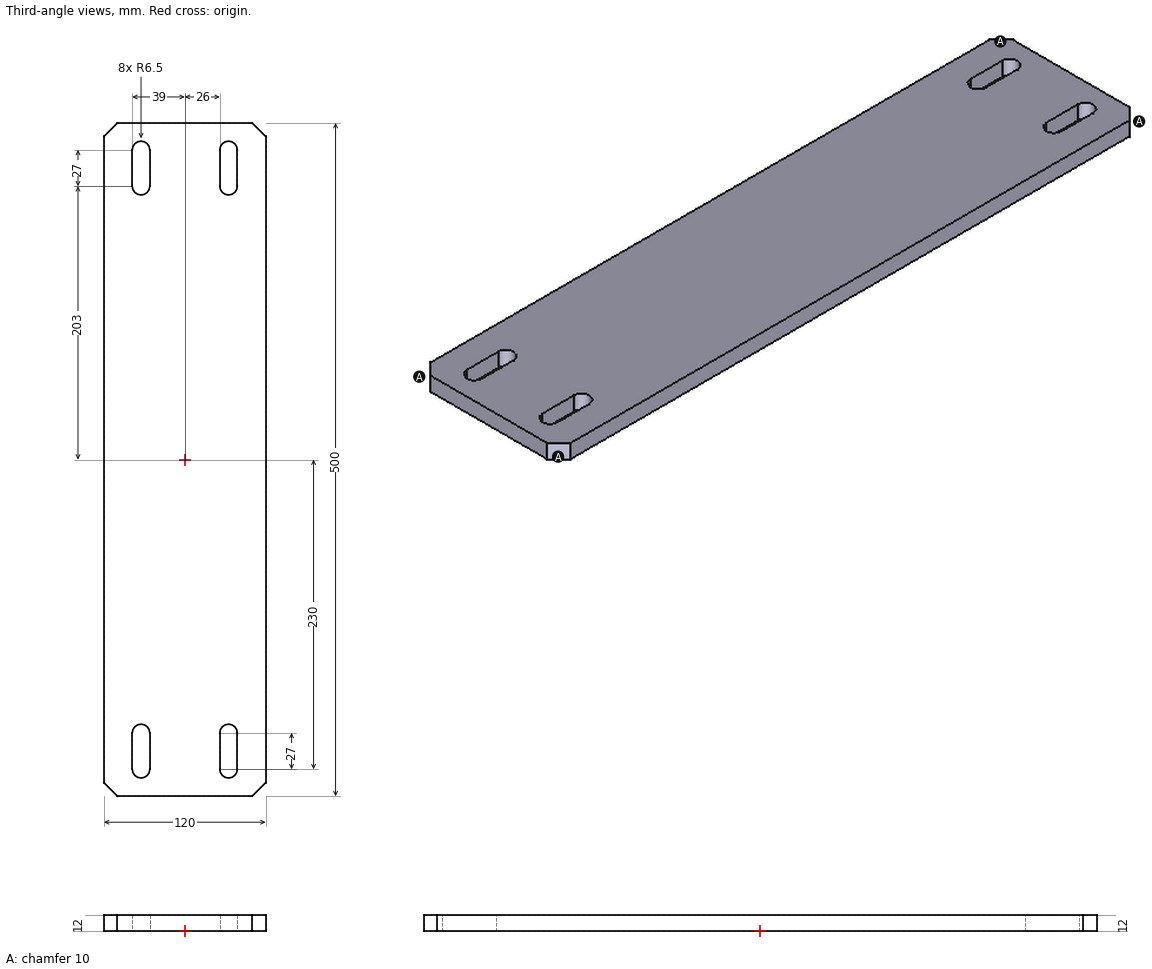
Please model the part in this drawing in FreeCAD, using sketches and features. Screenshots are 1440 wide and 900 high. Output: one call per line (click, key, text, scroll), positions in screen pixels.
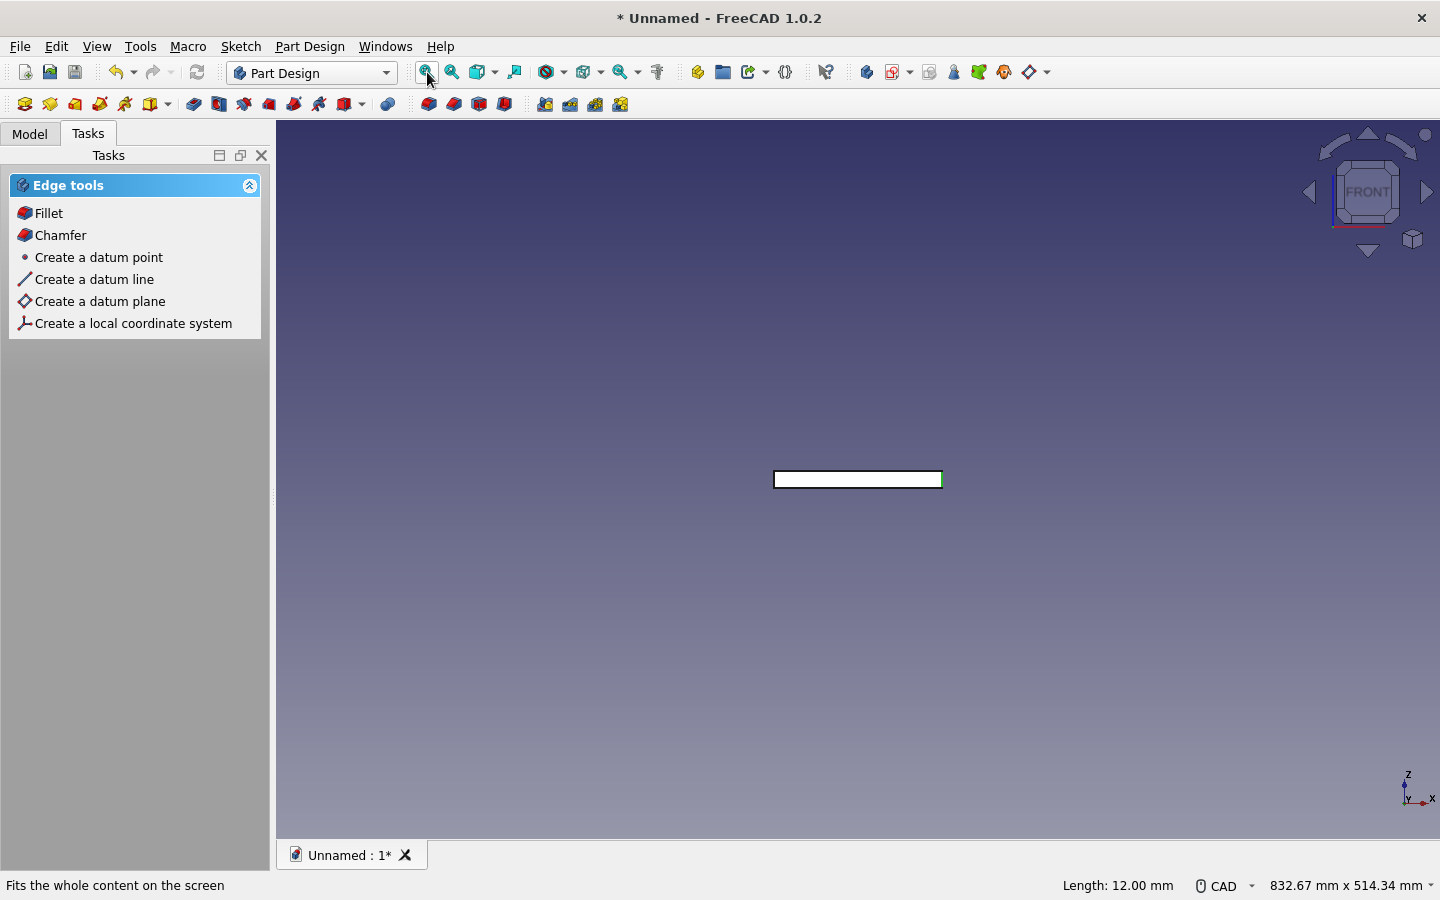
click(774, 479, ctrl)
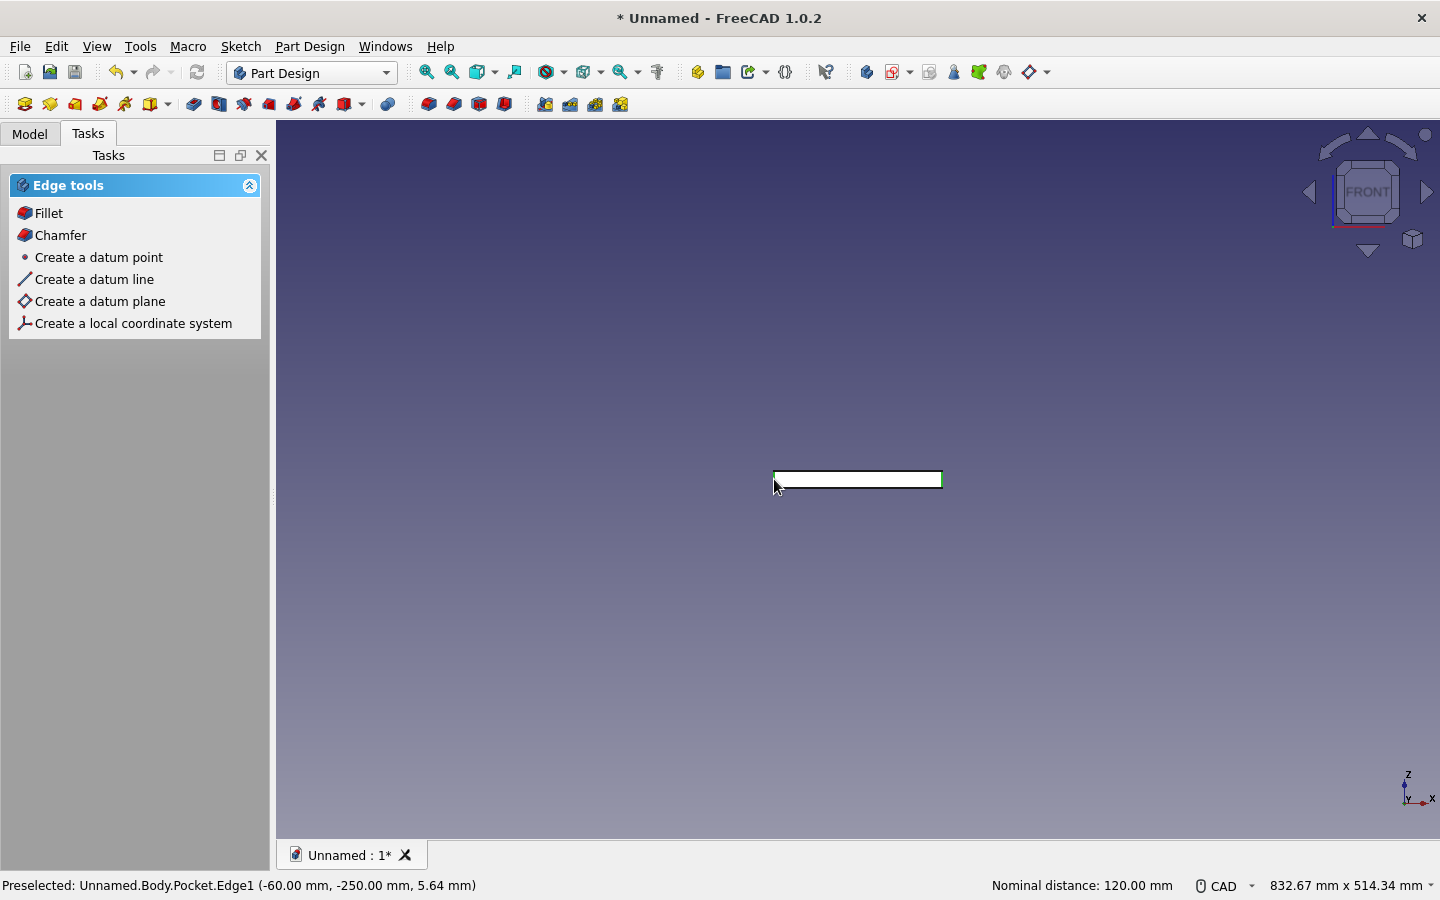
scroll(774, 479, up, 5)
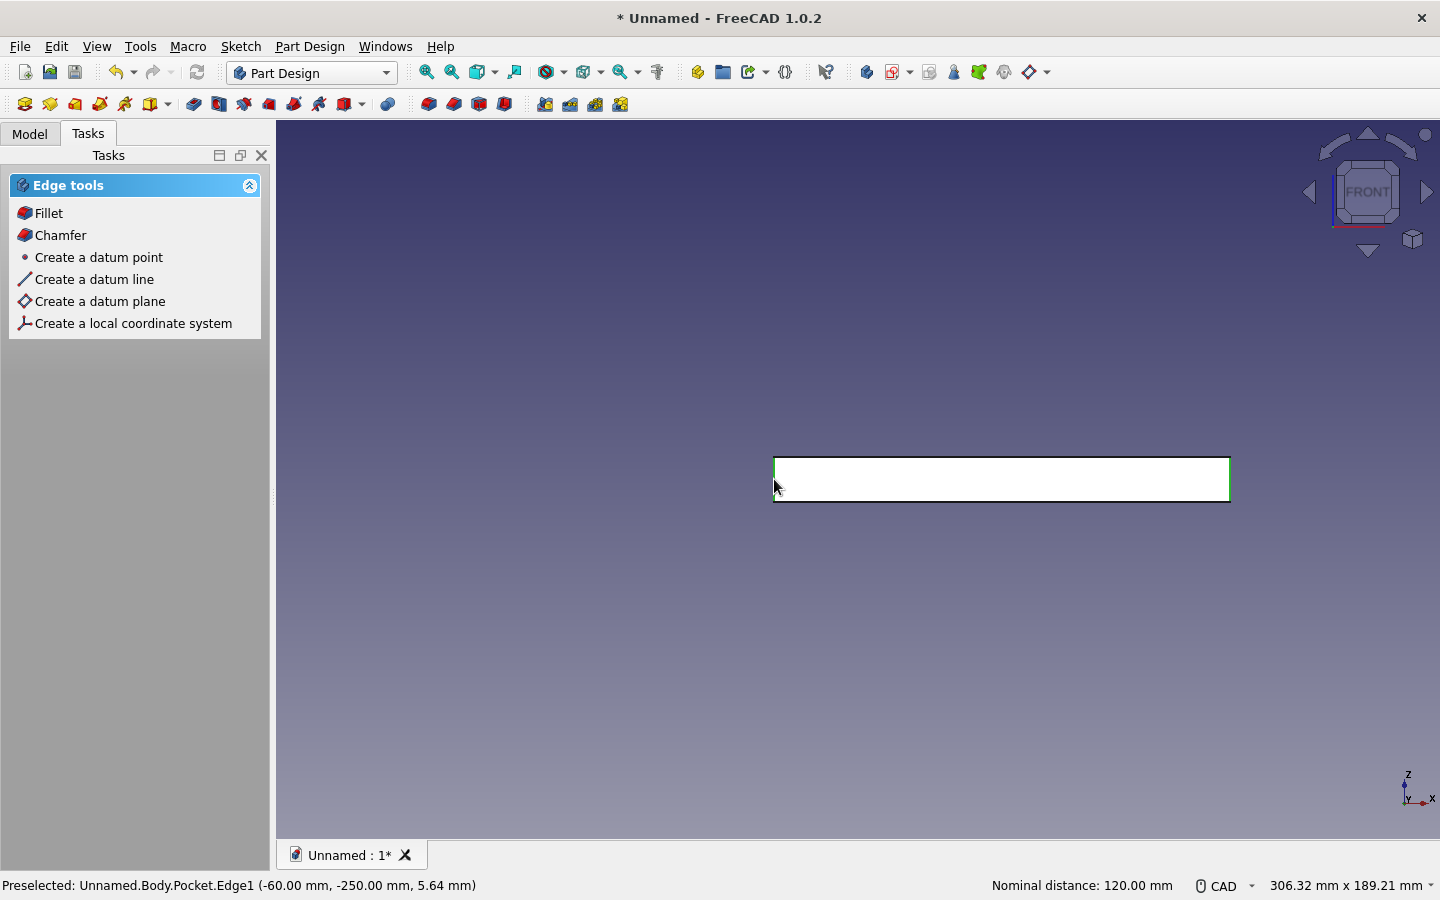
key(v)
key(f)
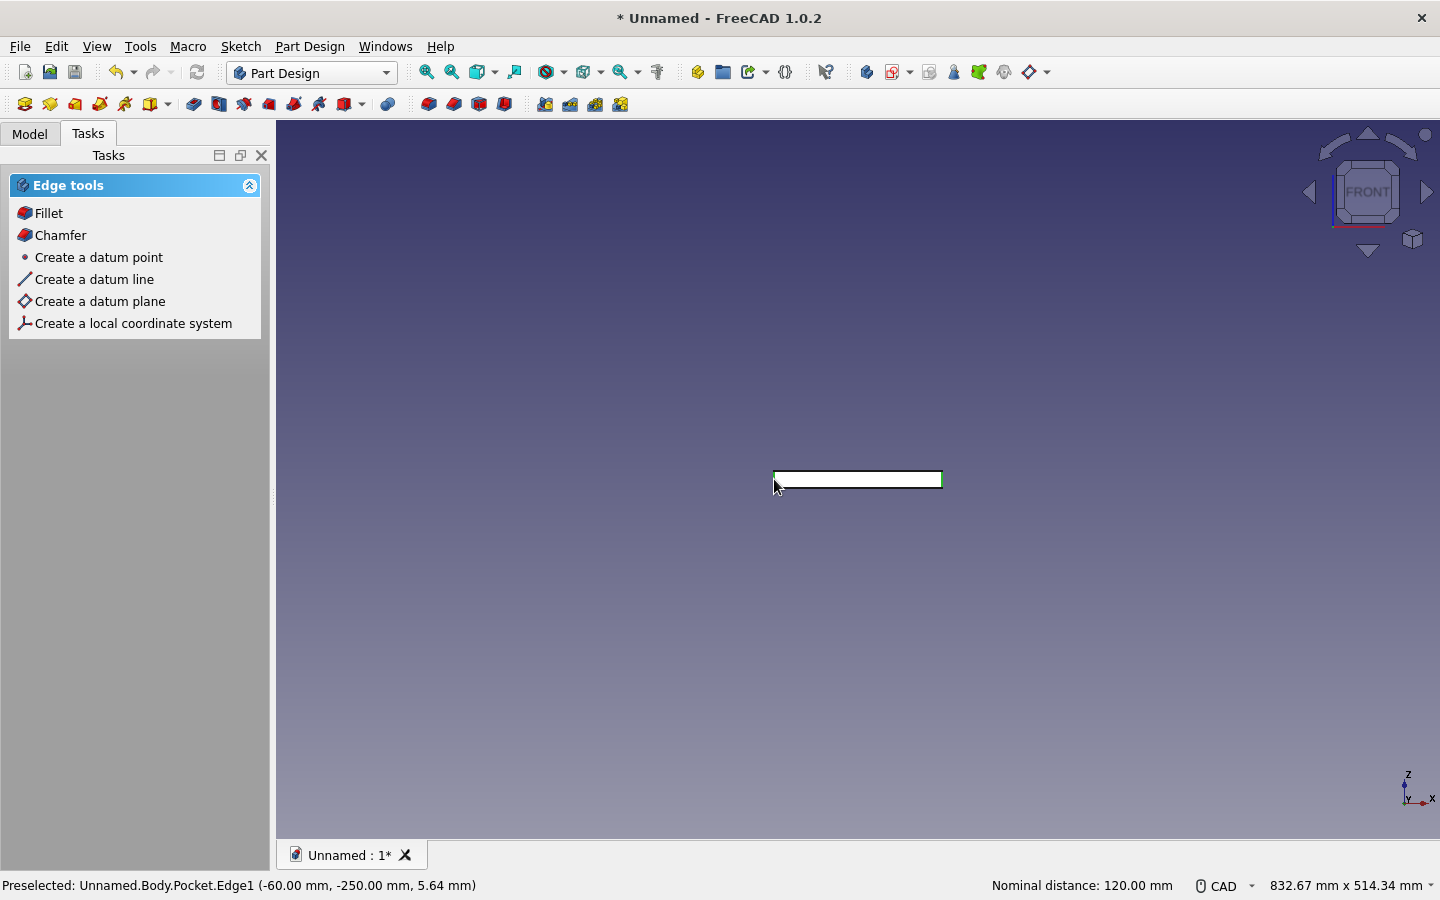
key(3)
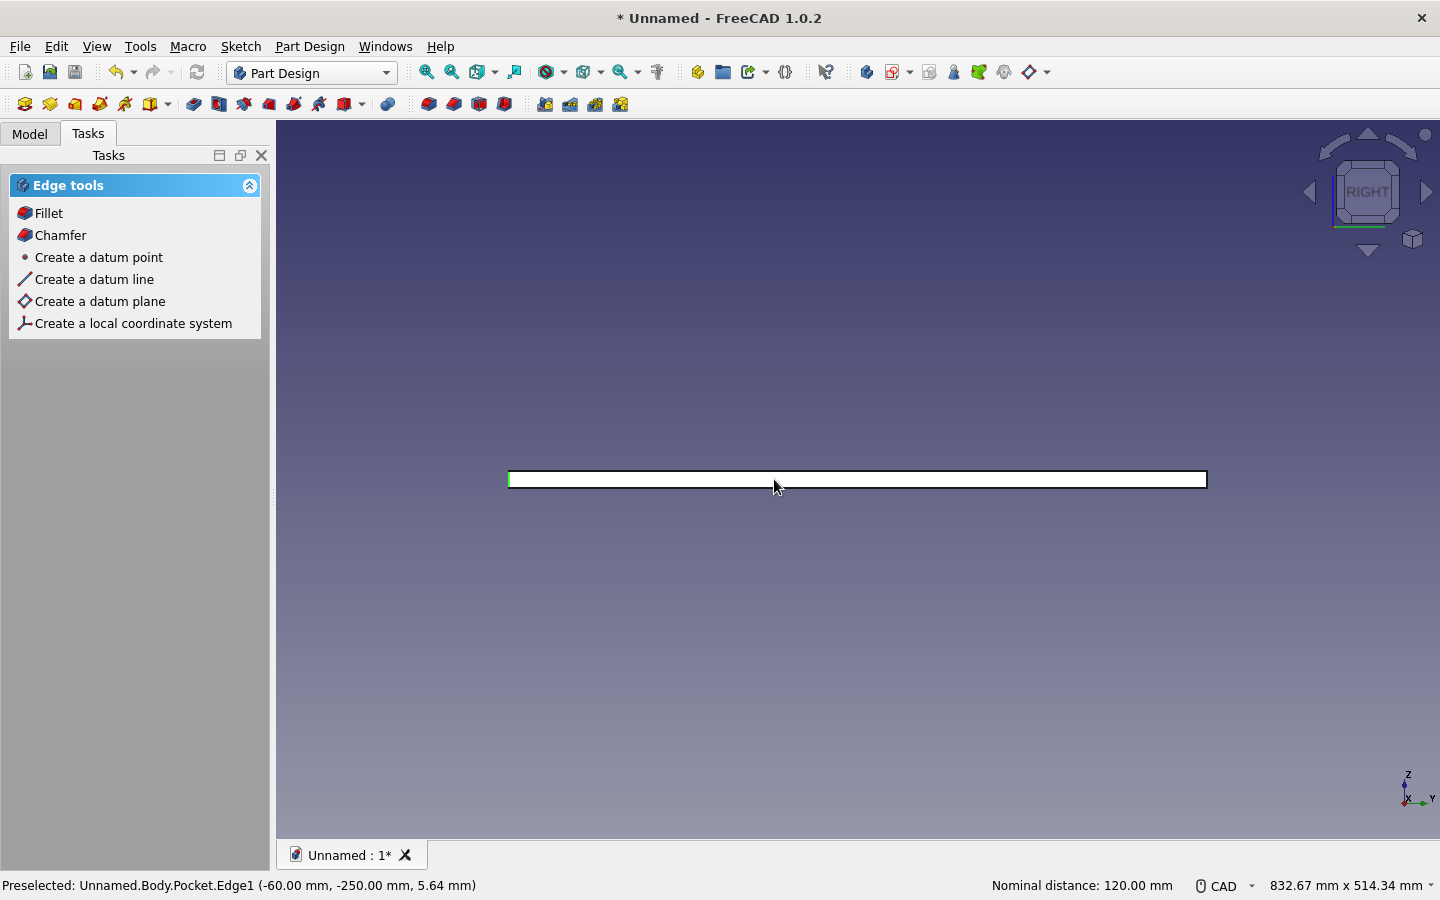
click(1207, 478, ctrl)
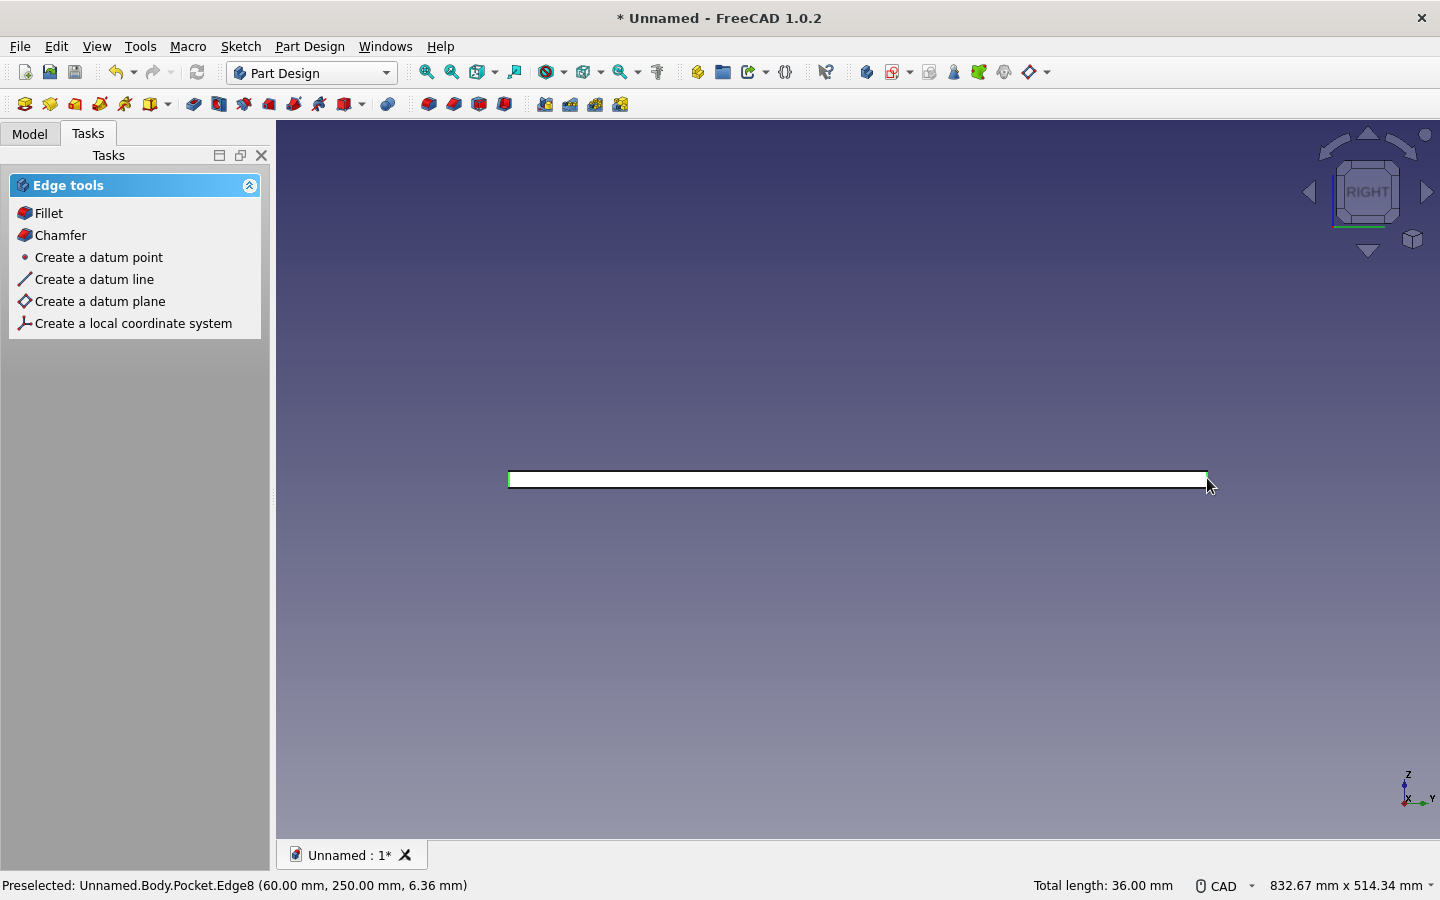
scroll(1207, 478, up, 5)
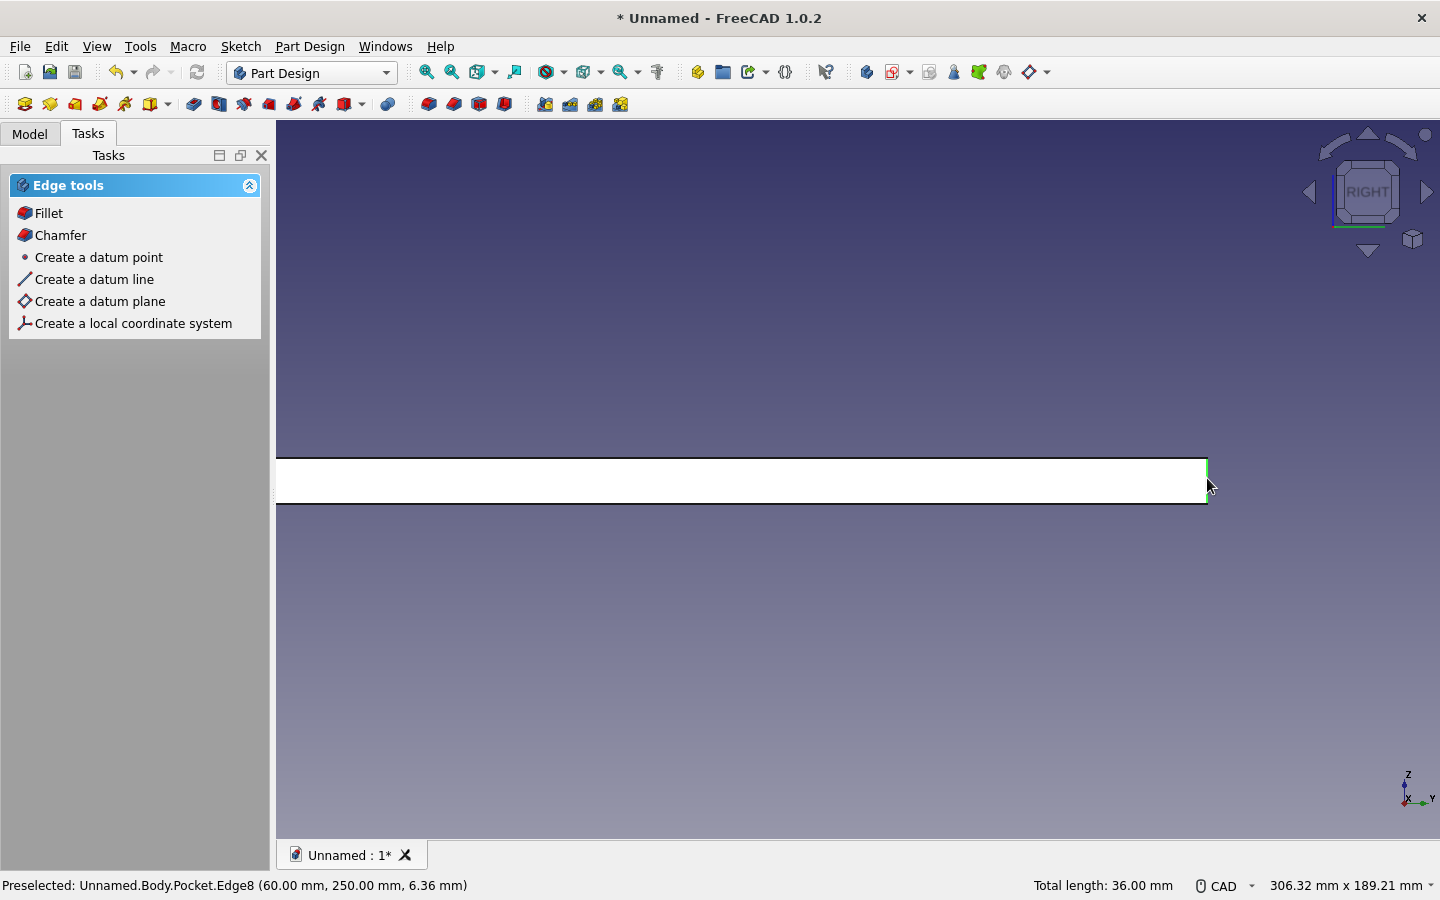
click(427, 72)